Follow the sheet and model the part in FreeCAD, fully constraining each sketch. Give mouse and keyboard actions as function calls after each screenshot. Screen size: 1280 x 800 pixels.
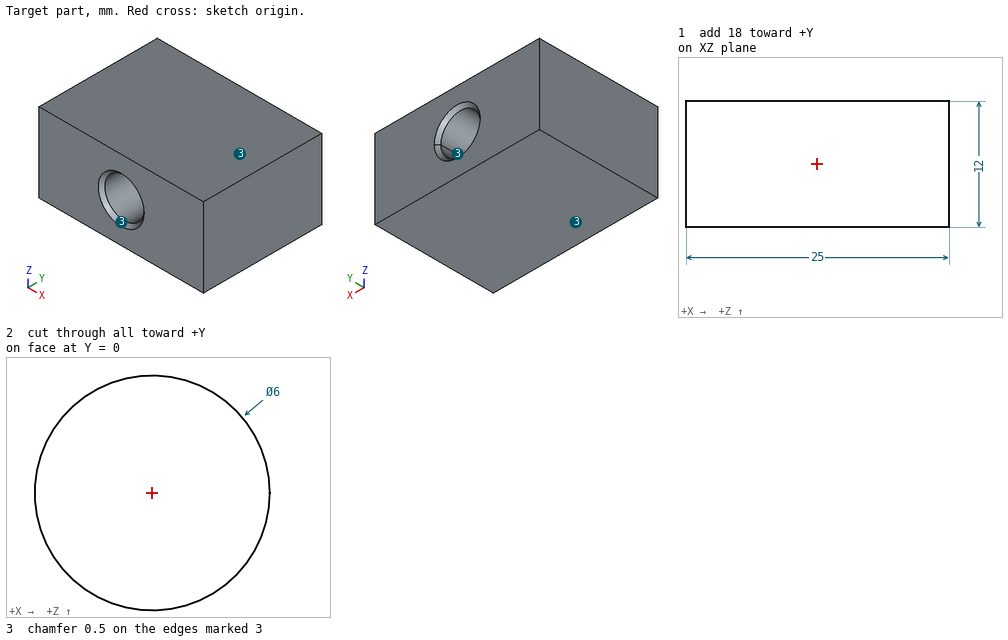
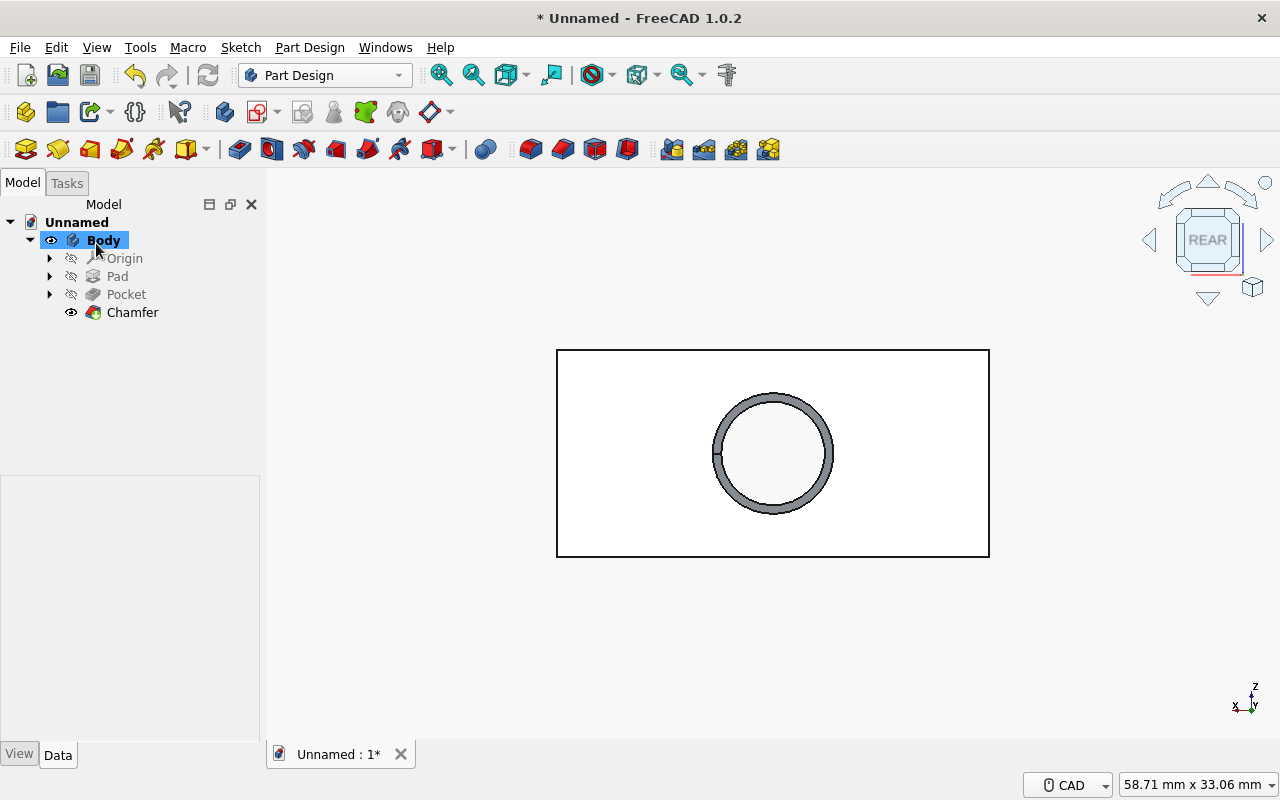
key(0)